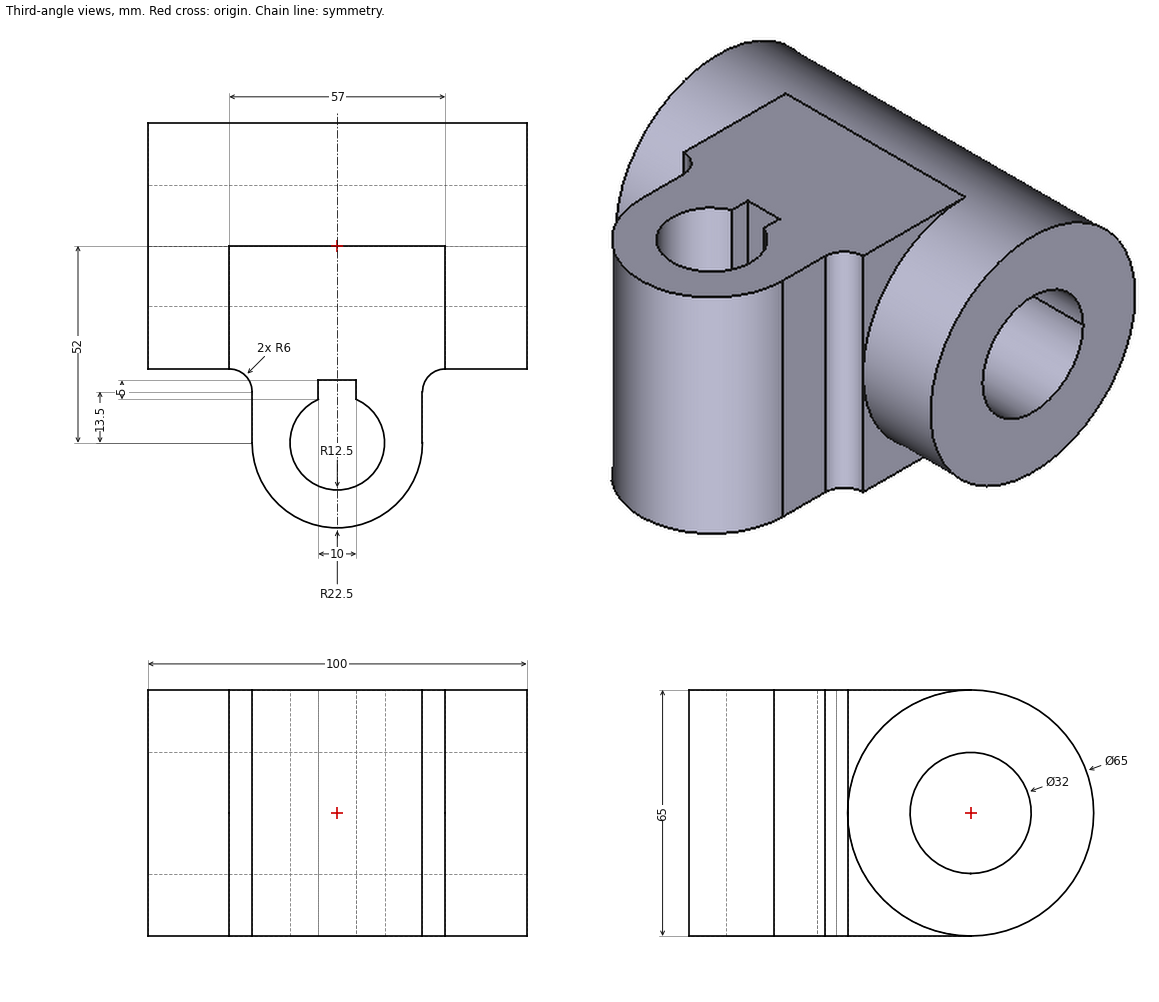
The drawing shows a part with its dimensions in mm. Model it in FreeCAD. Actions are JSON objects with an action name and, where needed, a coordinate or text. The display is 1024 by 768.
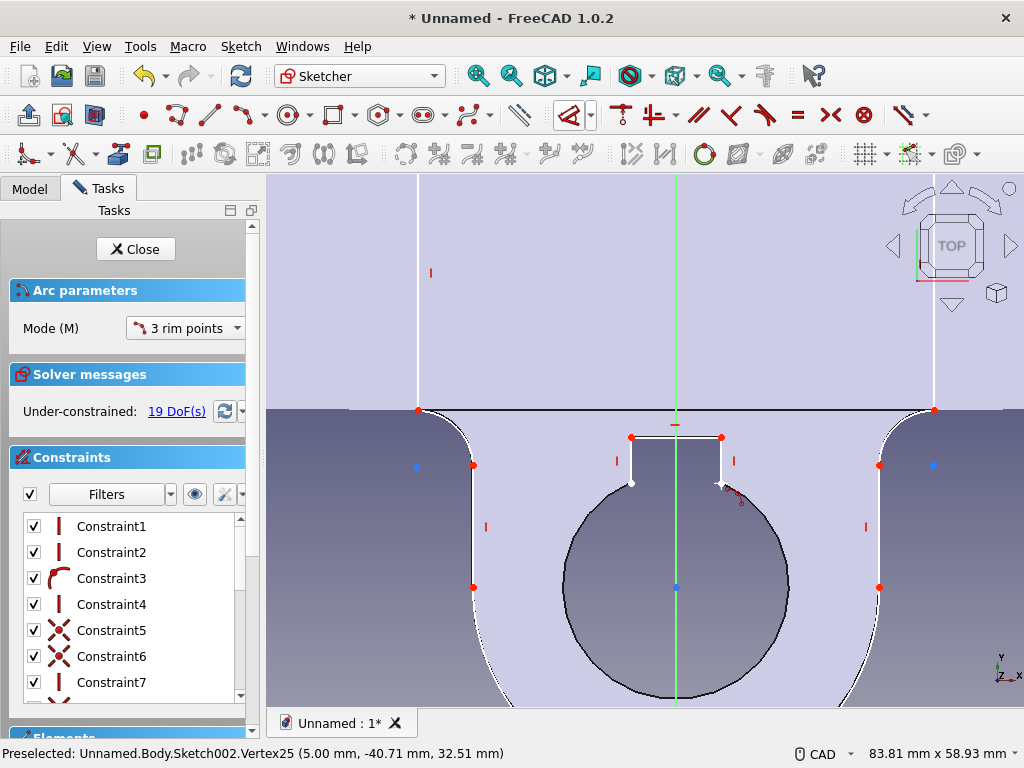
{"action": "left_click", "coordinate": [721, 484]}
{"action": "left_click", "coordinate": [631, 484]}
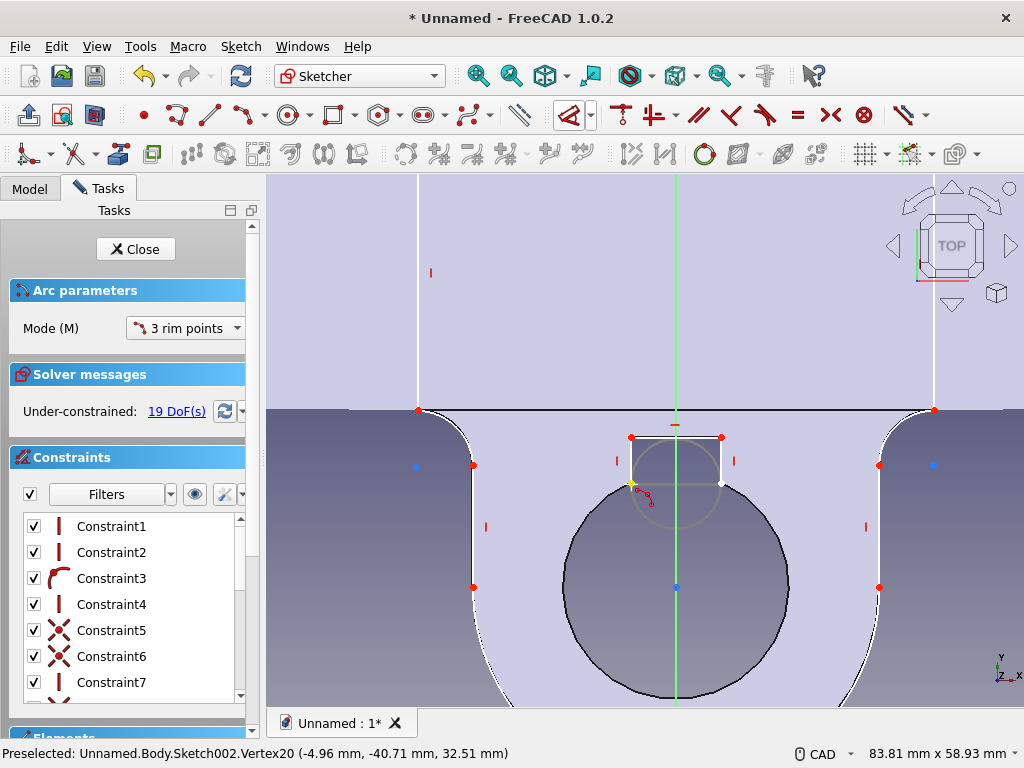
{"action": "scroll", "coordinate": [456, 426], "scroll_direction": "down", "scroll_amount": 3}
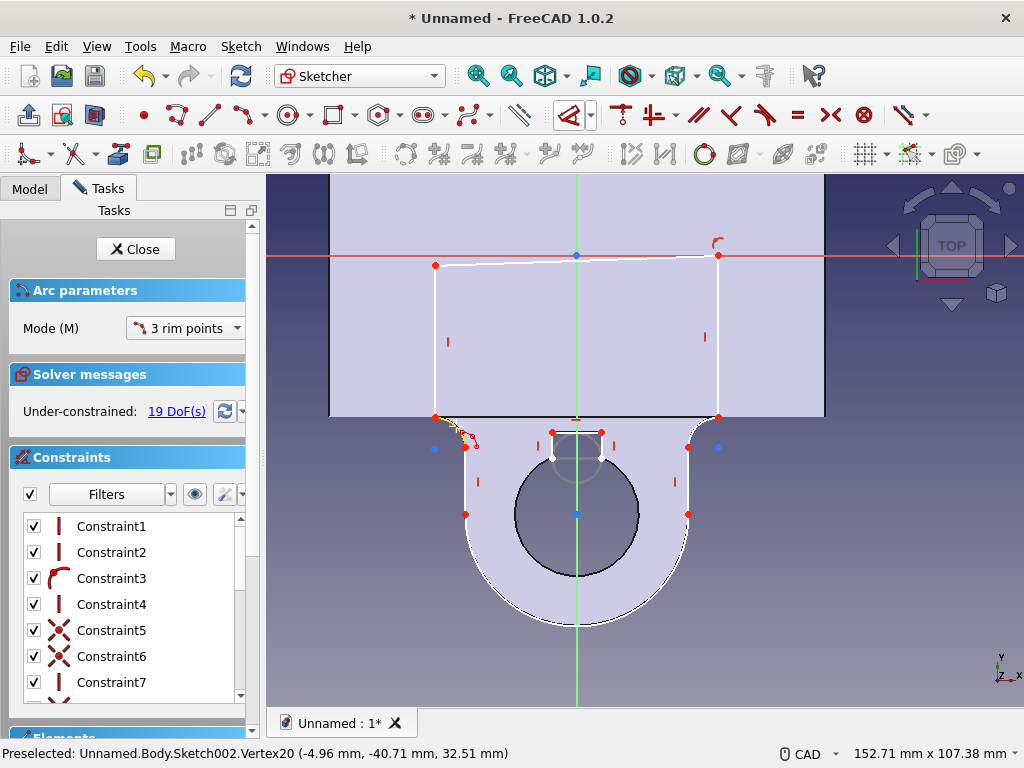
{"action": "left_click", "coordinate": [545, 567]}
{"action": "key", "text": "Escape"}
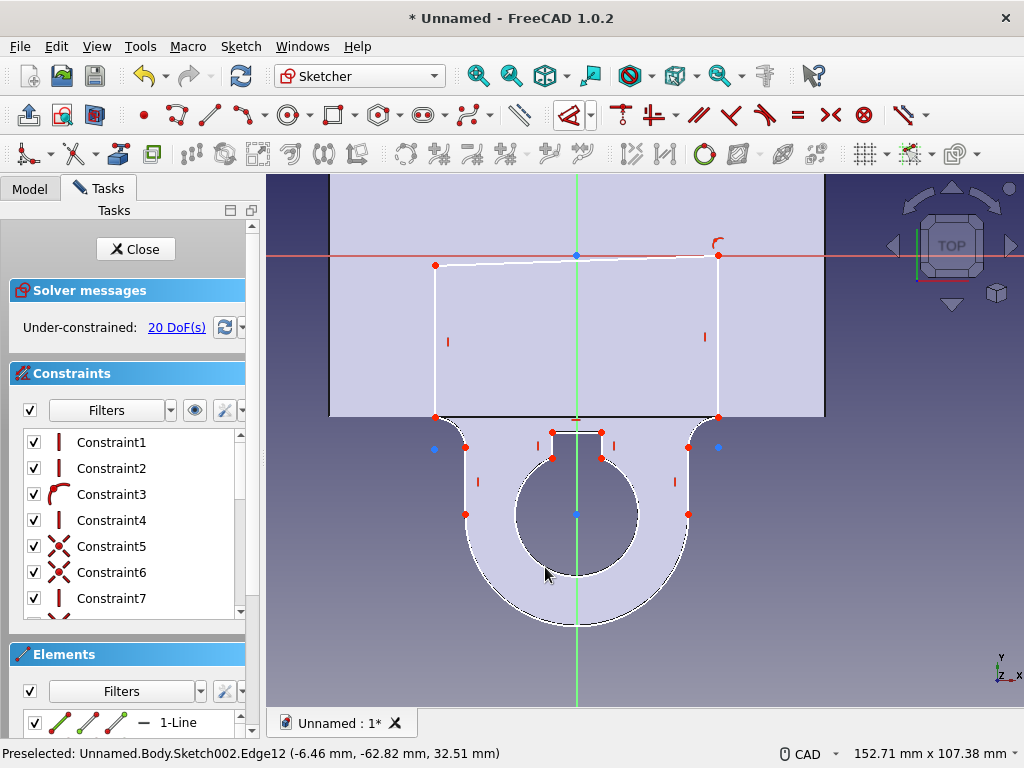
{"action": "left_click", "coordinate": [465, 468]}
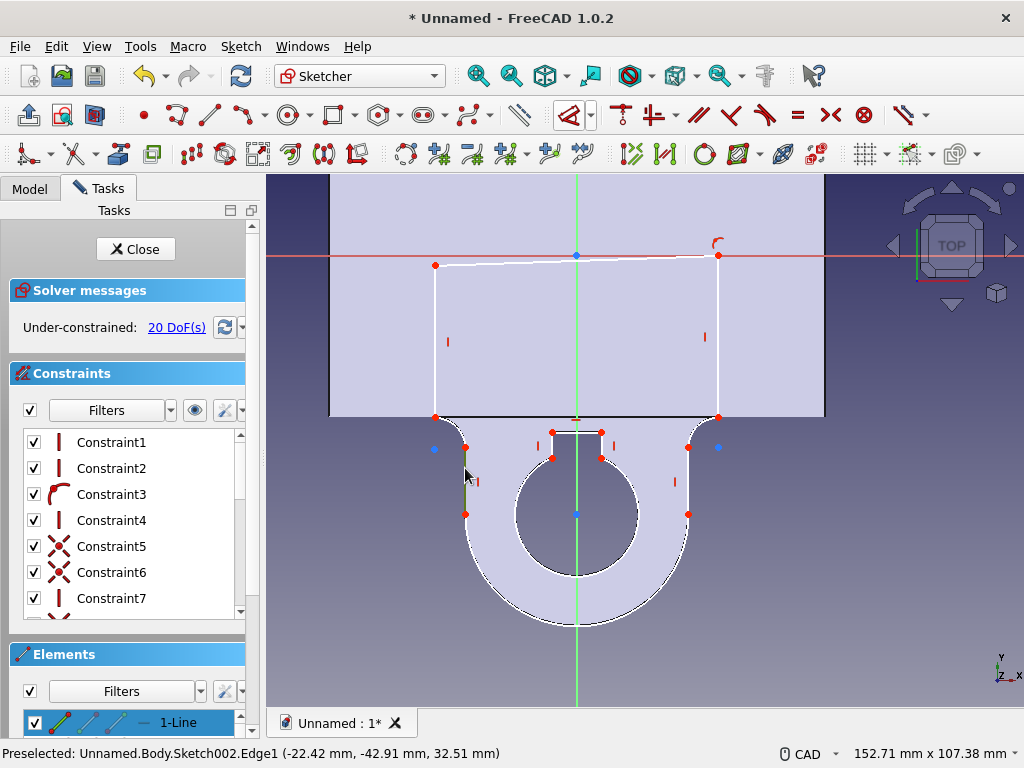
{"action": "left_click", "coordinate": [511, 605]}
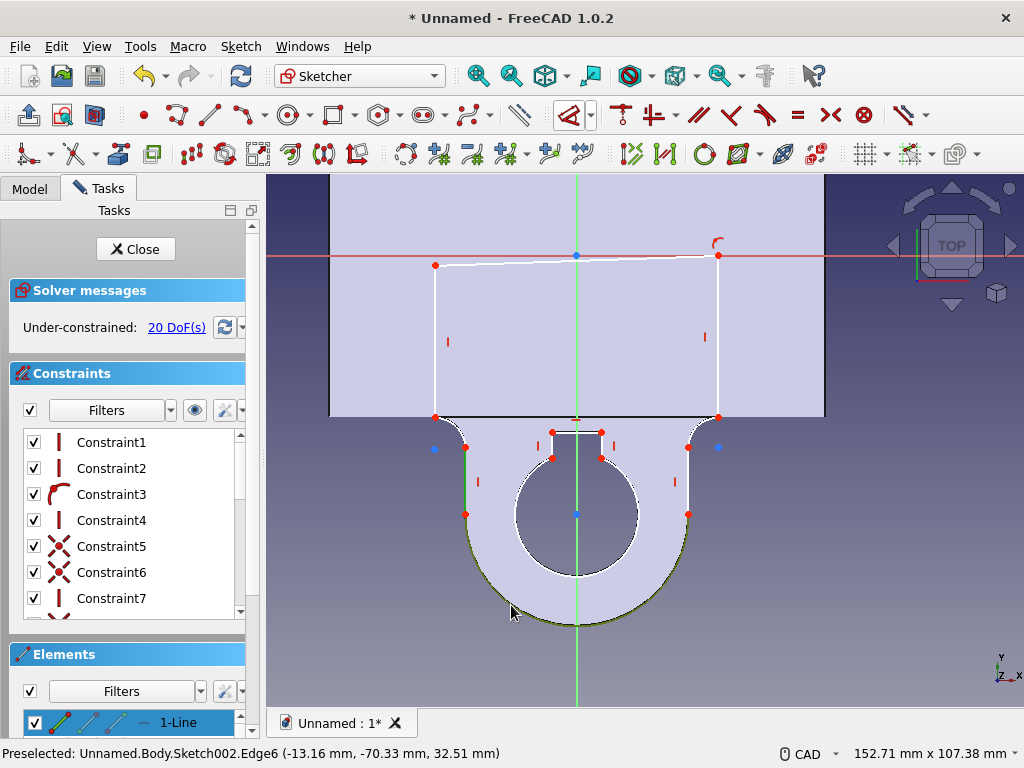
{"action": "key", "text": "t"}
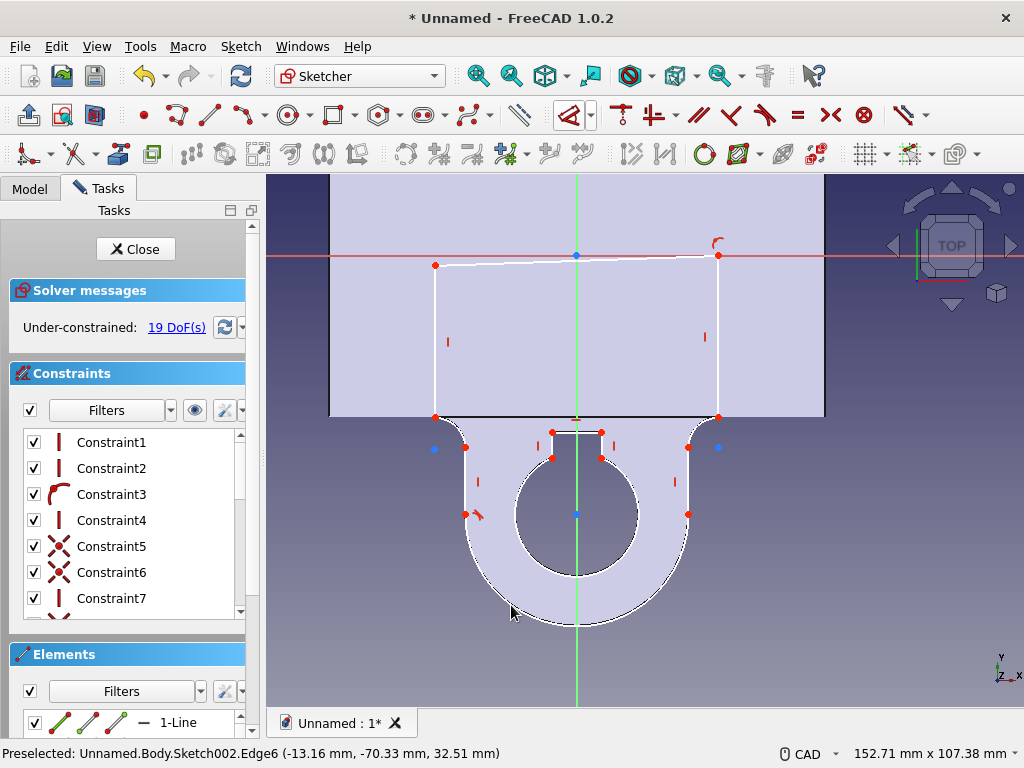
{"action": "left_click", "coordinate": [465, 468]}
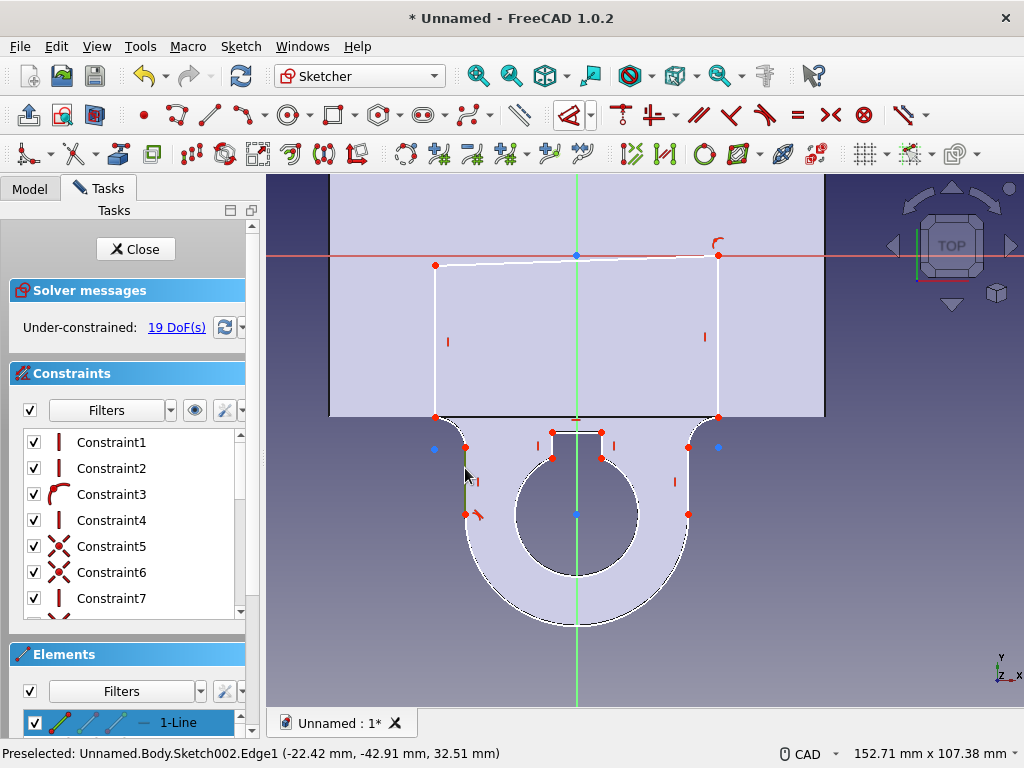
{"action": "left_click", "coordinate": [462, 434]}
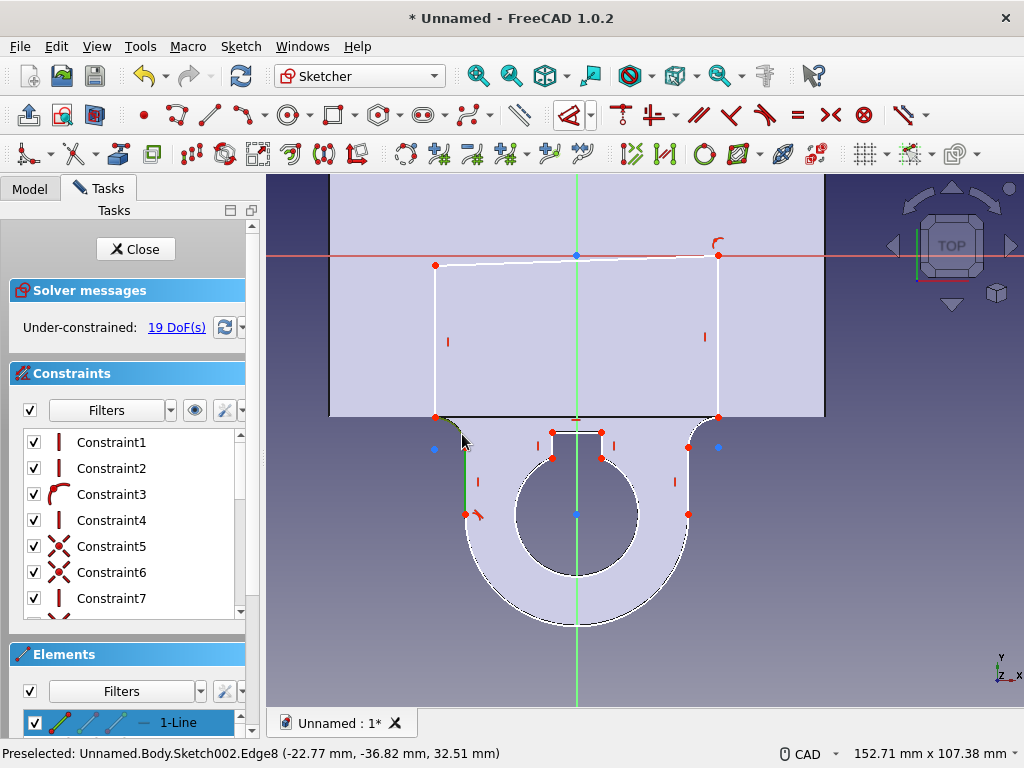
{"action": "key", "text": "t"}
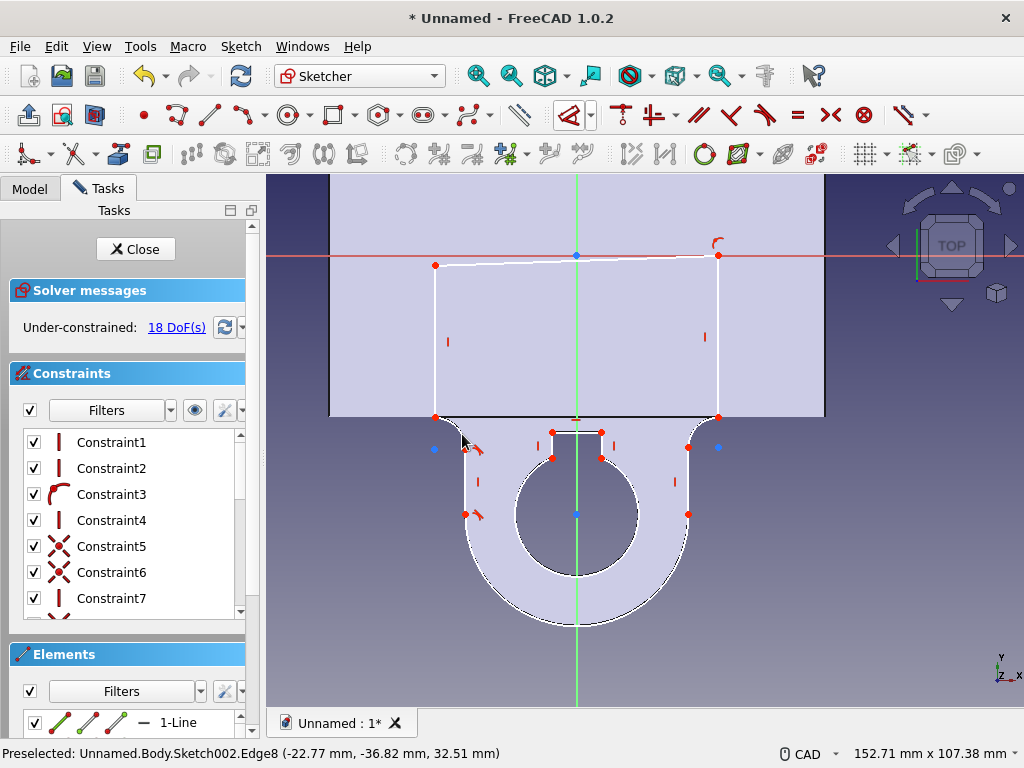
{"action": "left_click", "coordinate": [688, 495]}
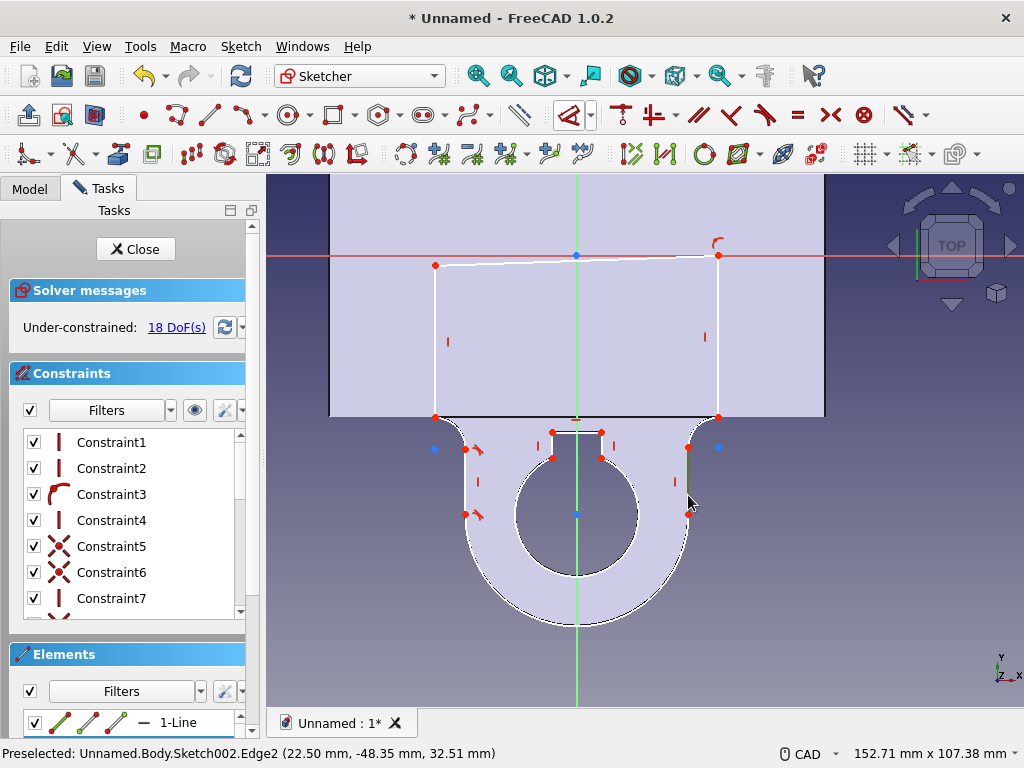
{"action": "left_click", "coordinate": [511, 605]}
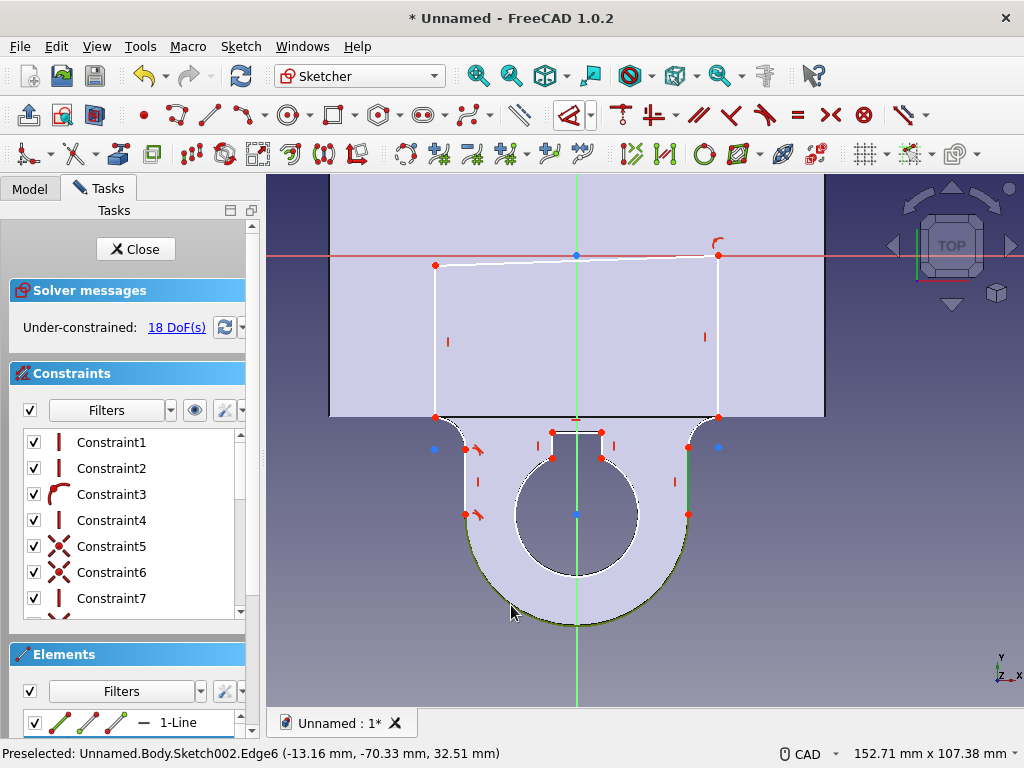
{"action": "left_click", "coordinate": [765, 116]}